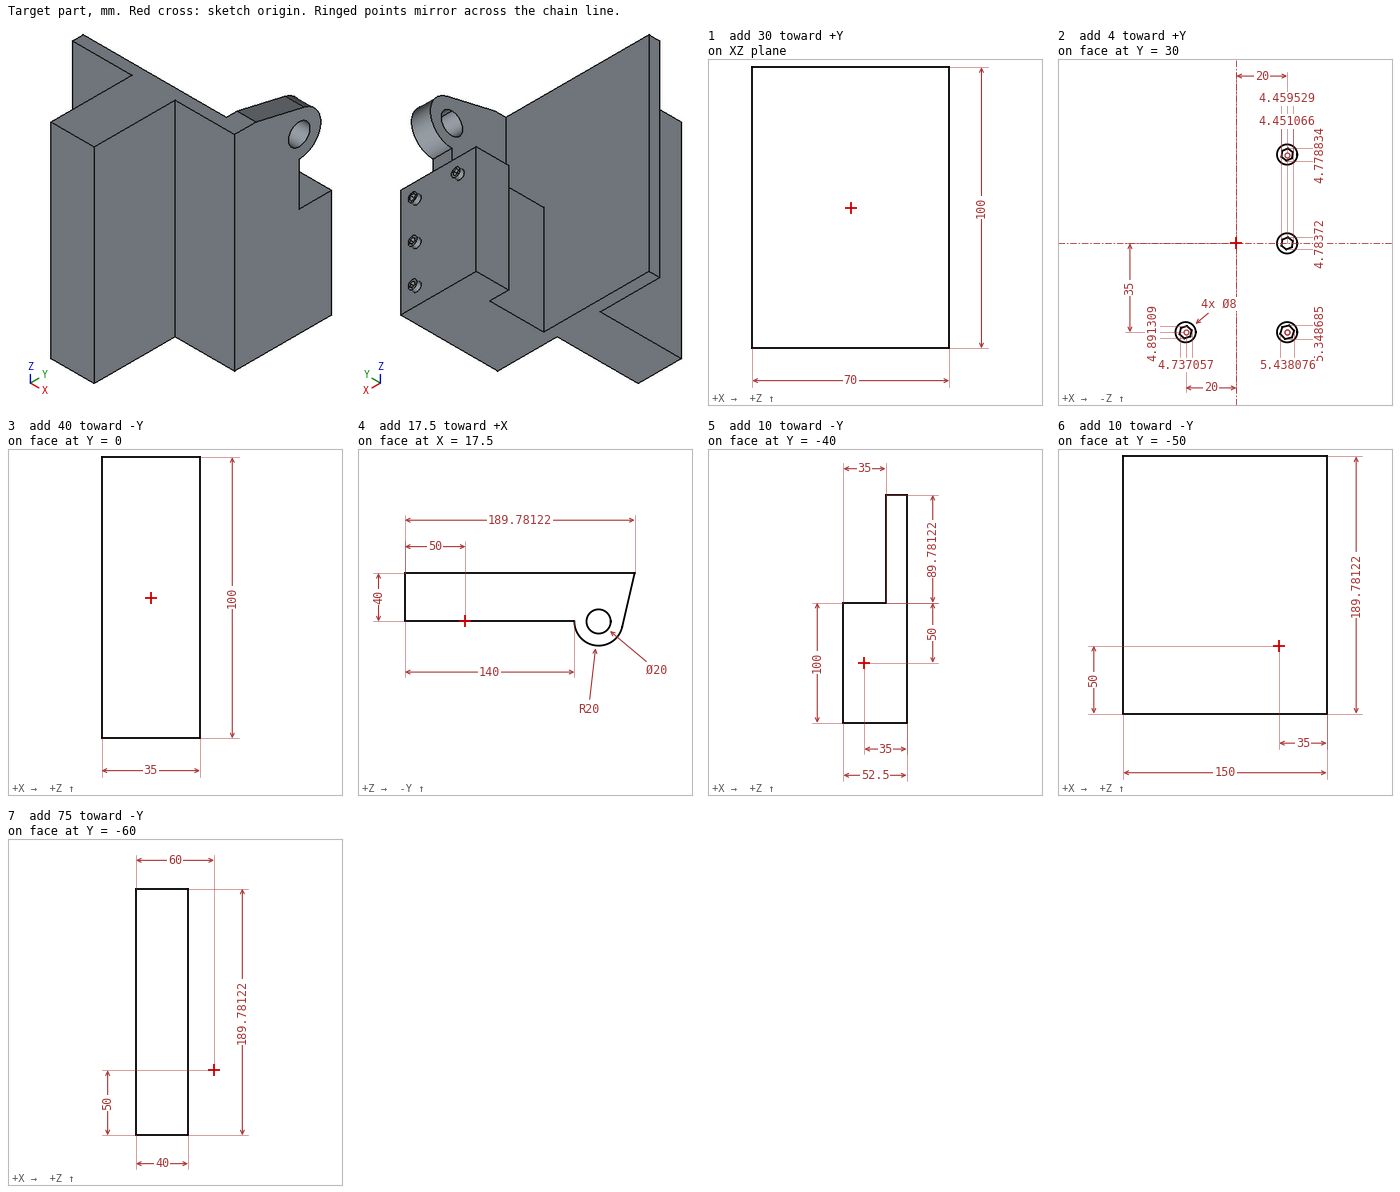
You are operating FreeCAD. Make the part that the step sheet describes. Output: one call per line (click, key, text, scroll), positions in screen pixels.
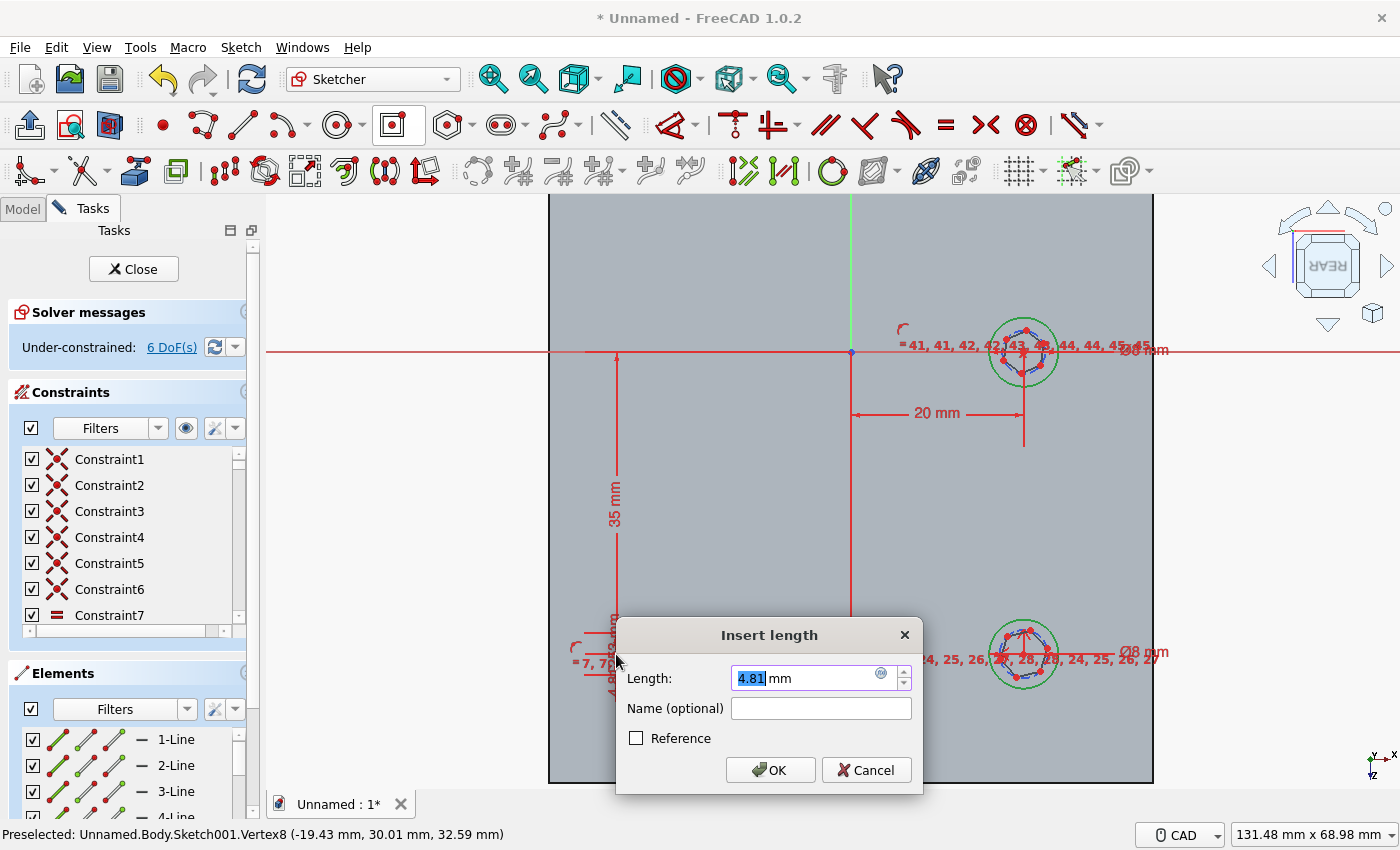
text(4.891309)
key(Return)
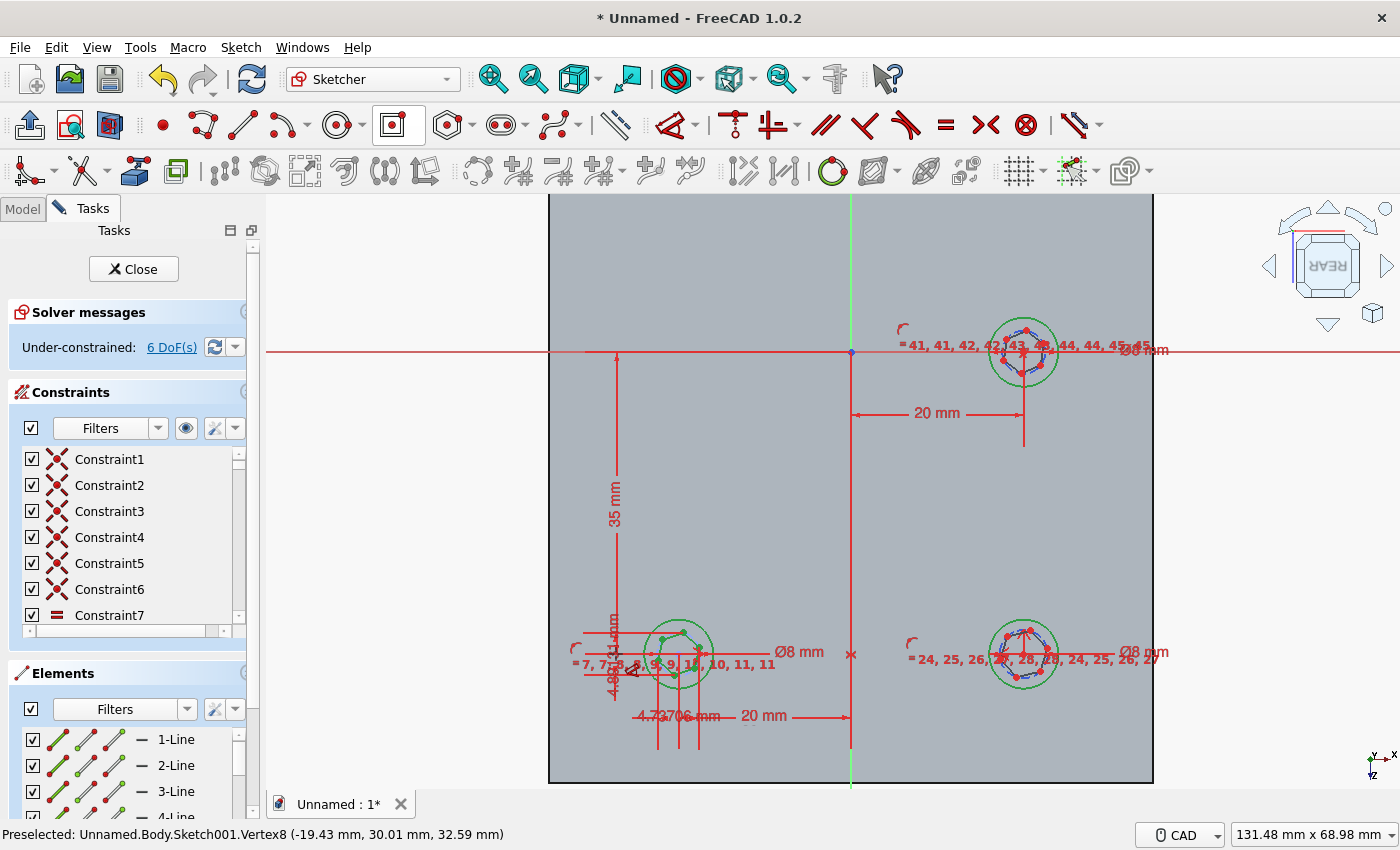
click(1000, 660)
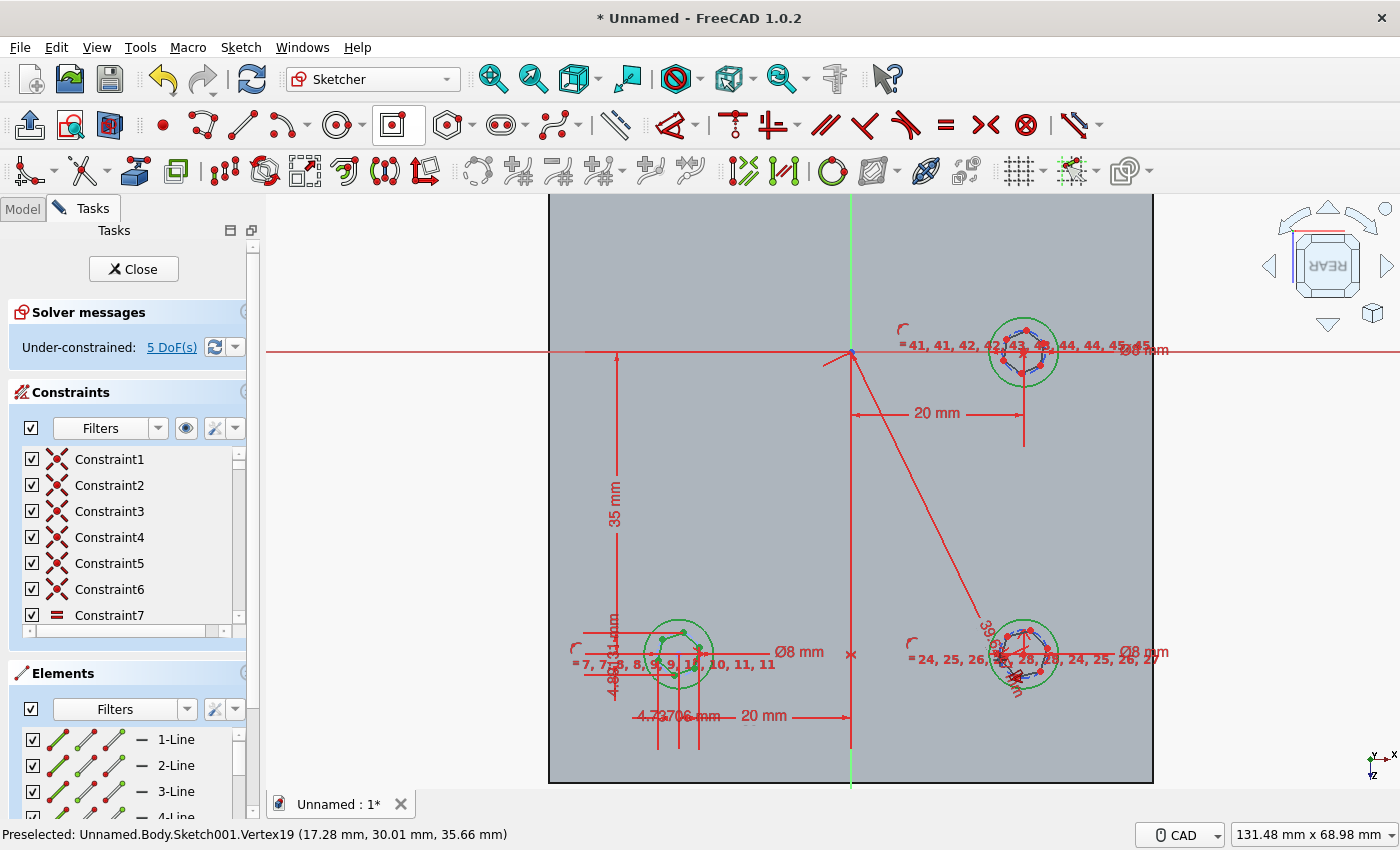
click(1047, 648)
click(1024, 718)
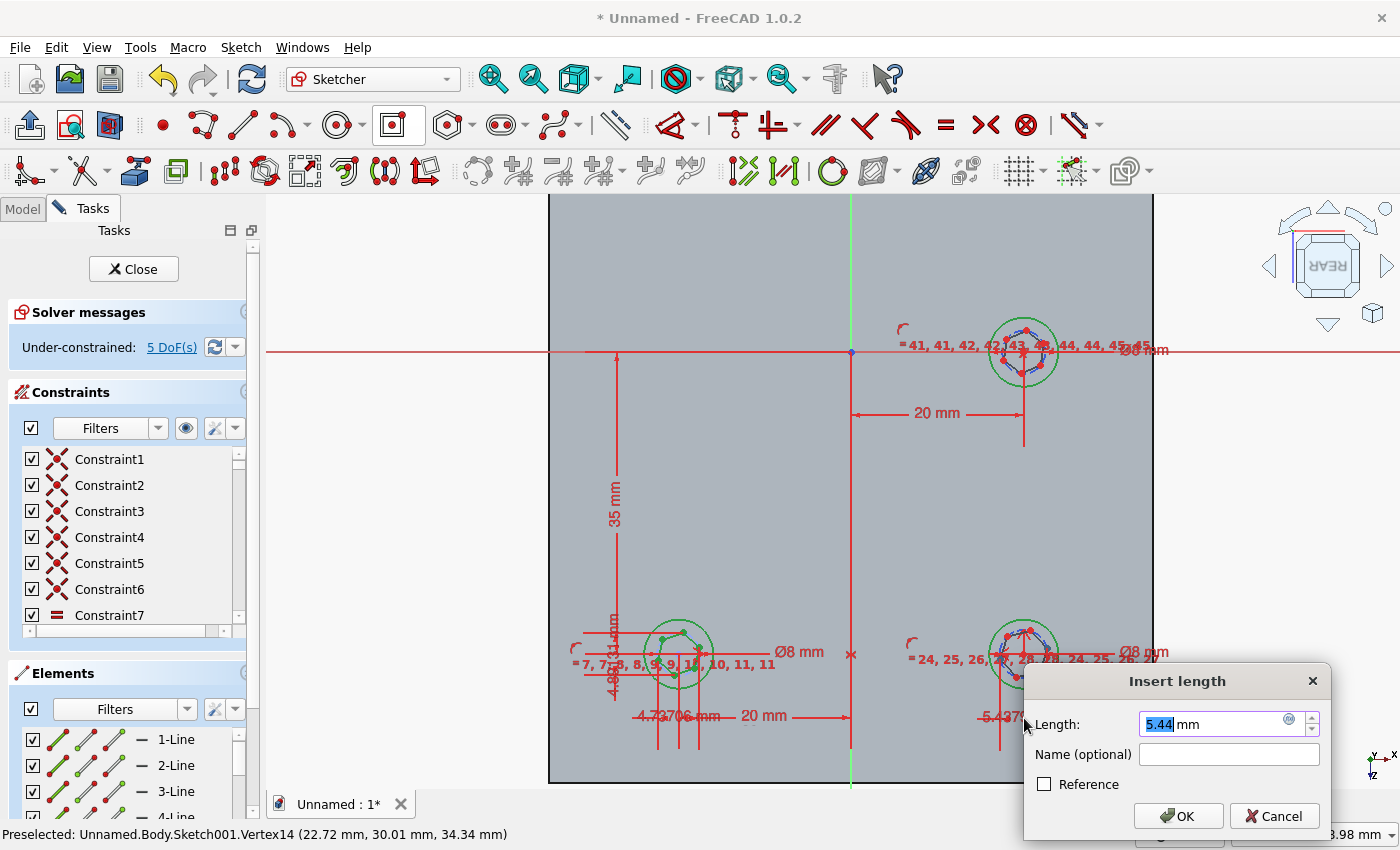
text(5.438076)
key(Return)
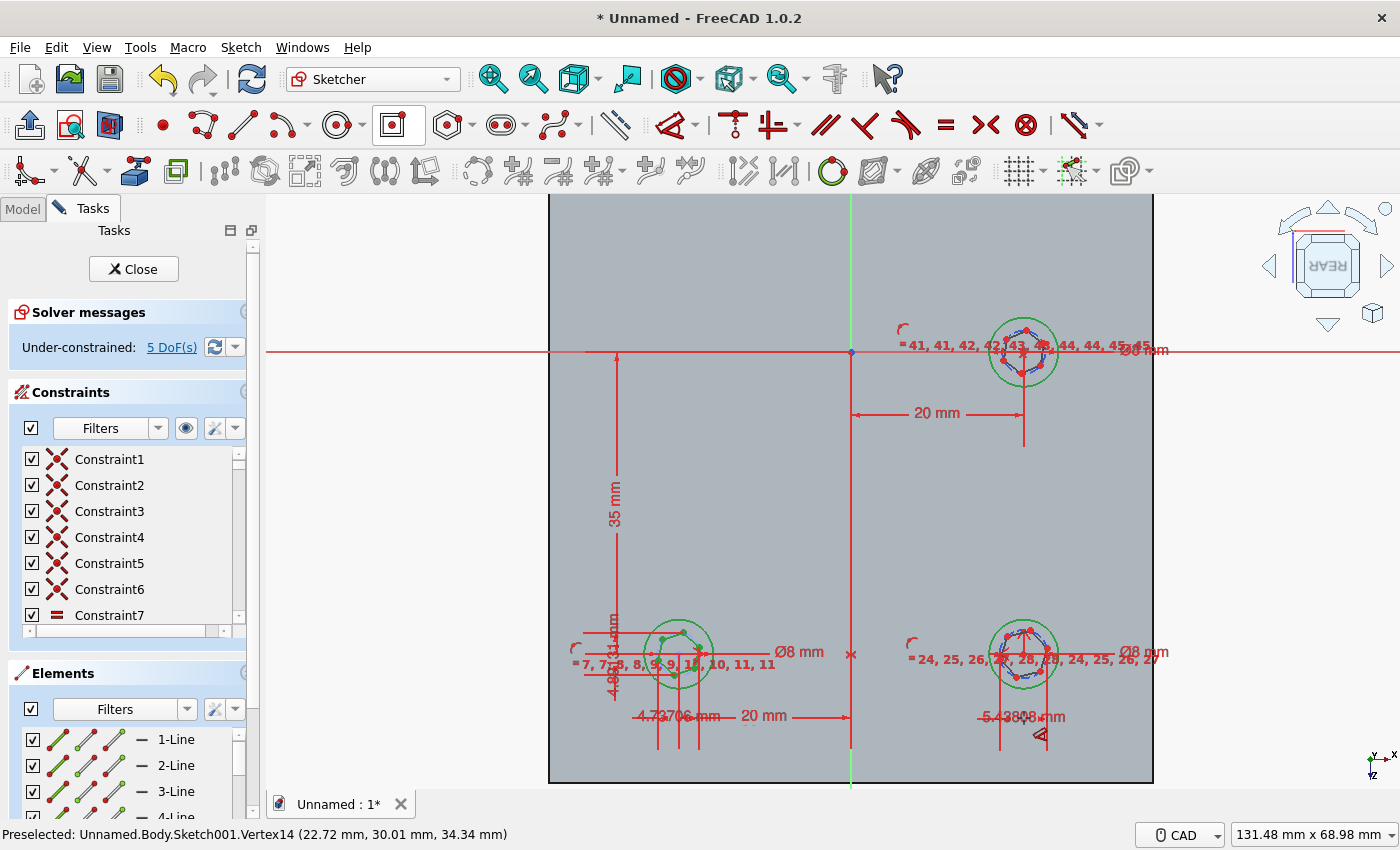
click(1017, 677)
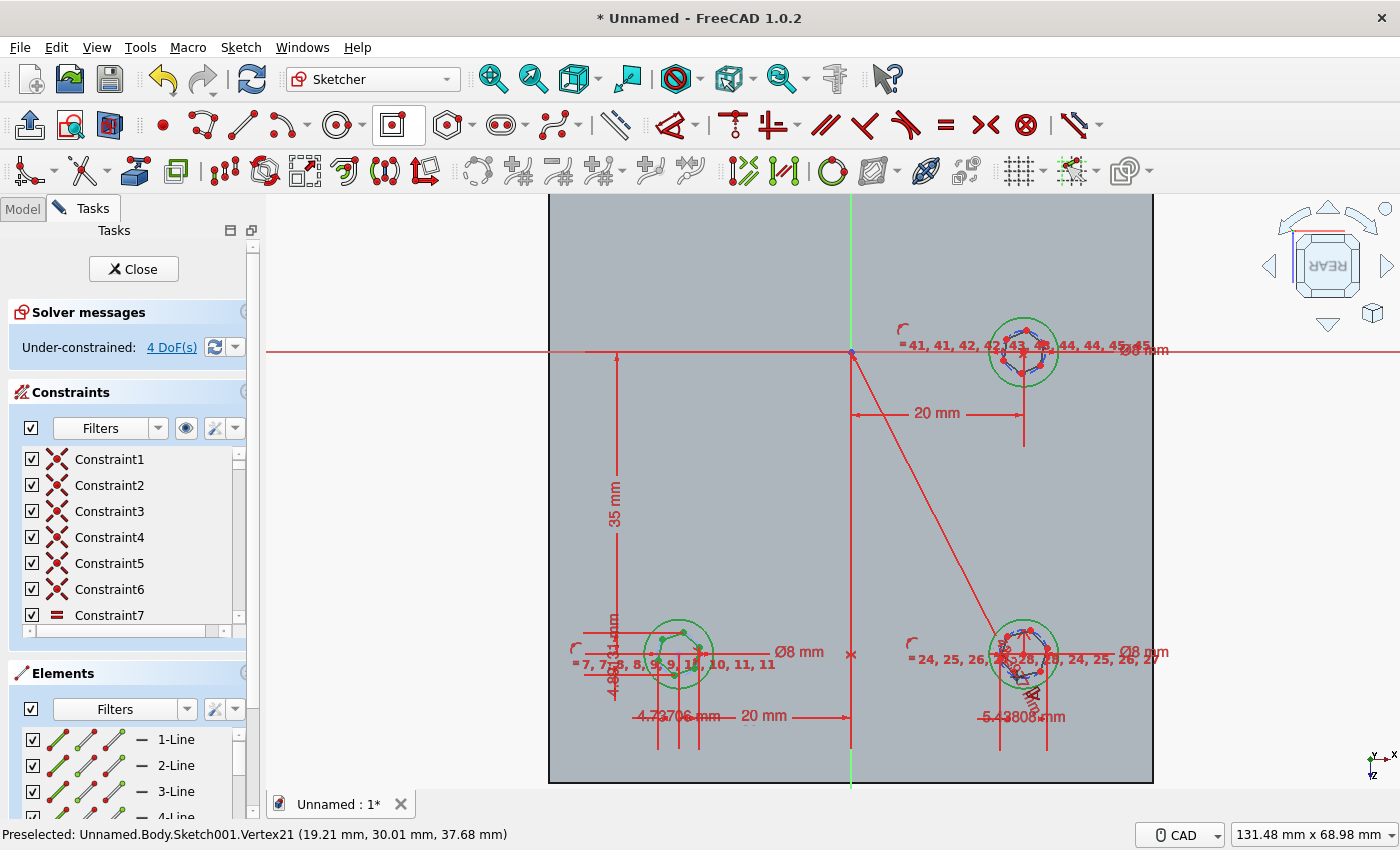
click(1031, 631)
click(1089, 654)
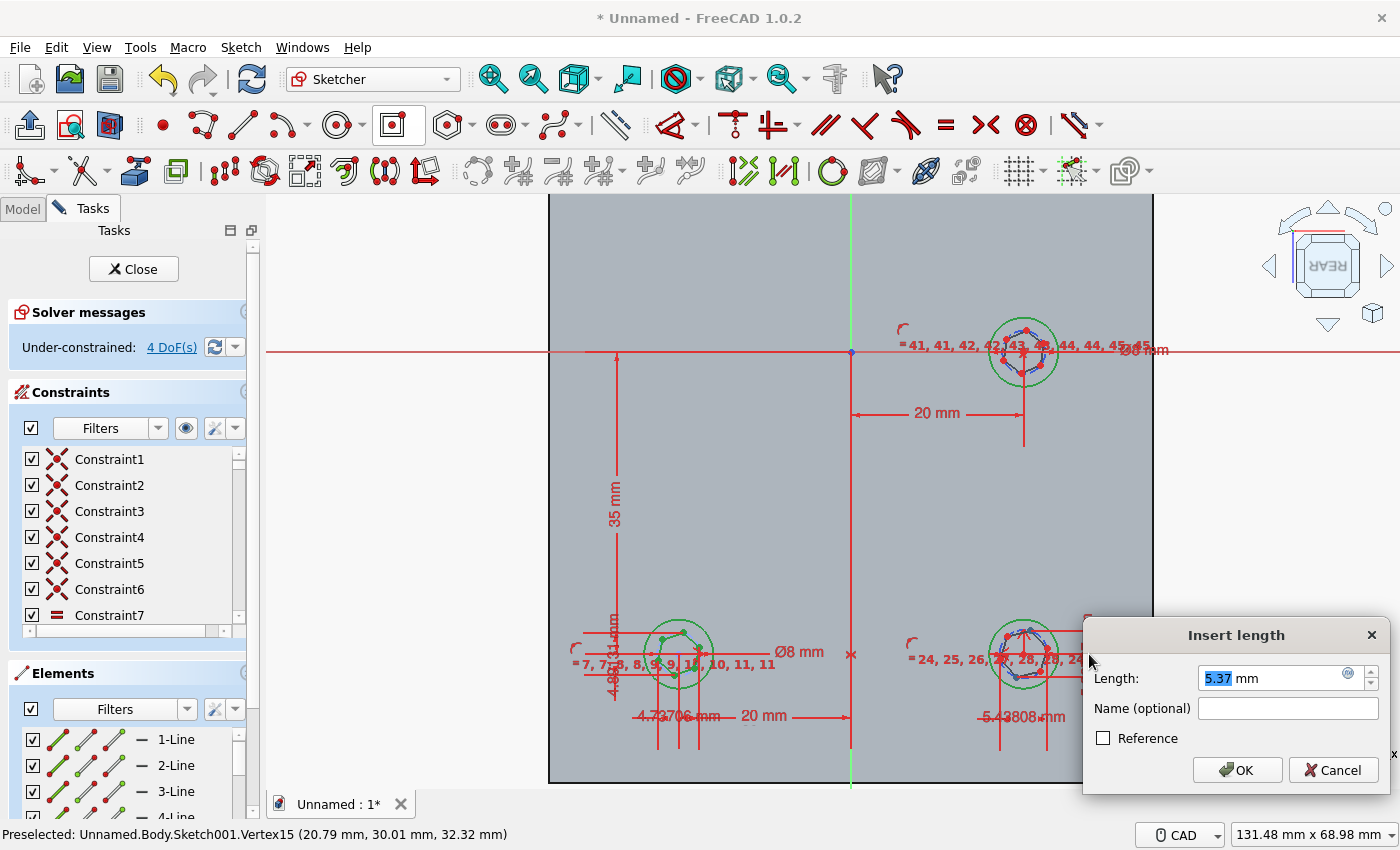
text(5.348685)
key(Return)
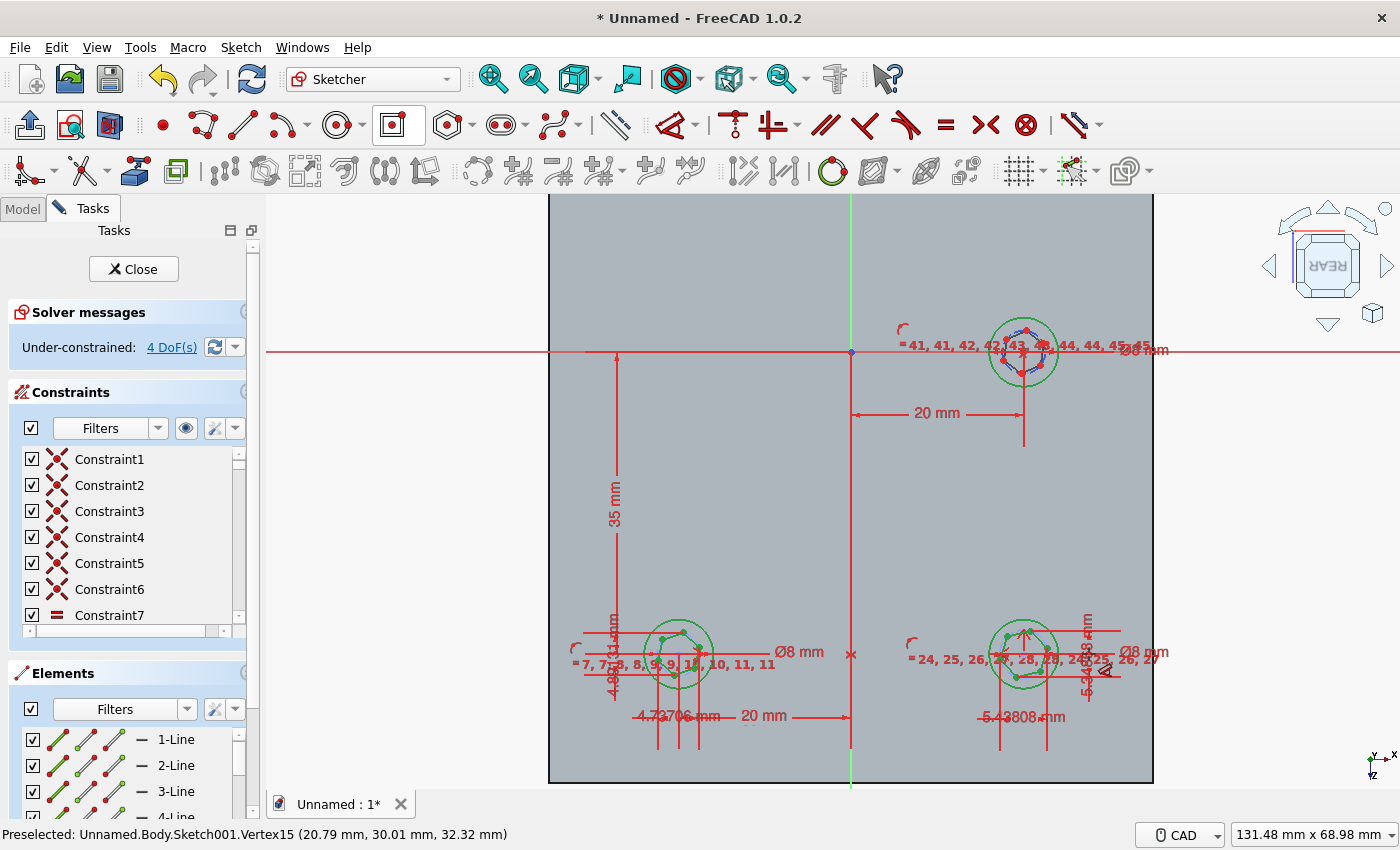
click(1004, 360)